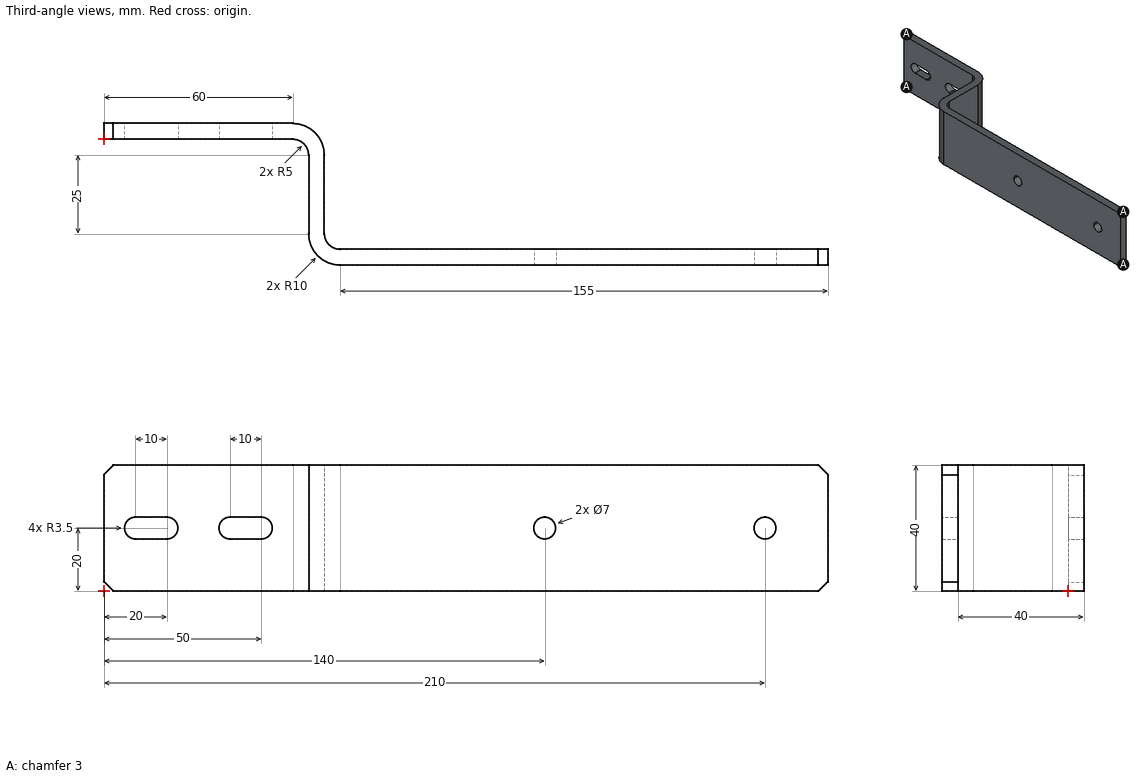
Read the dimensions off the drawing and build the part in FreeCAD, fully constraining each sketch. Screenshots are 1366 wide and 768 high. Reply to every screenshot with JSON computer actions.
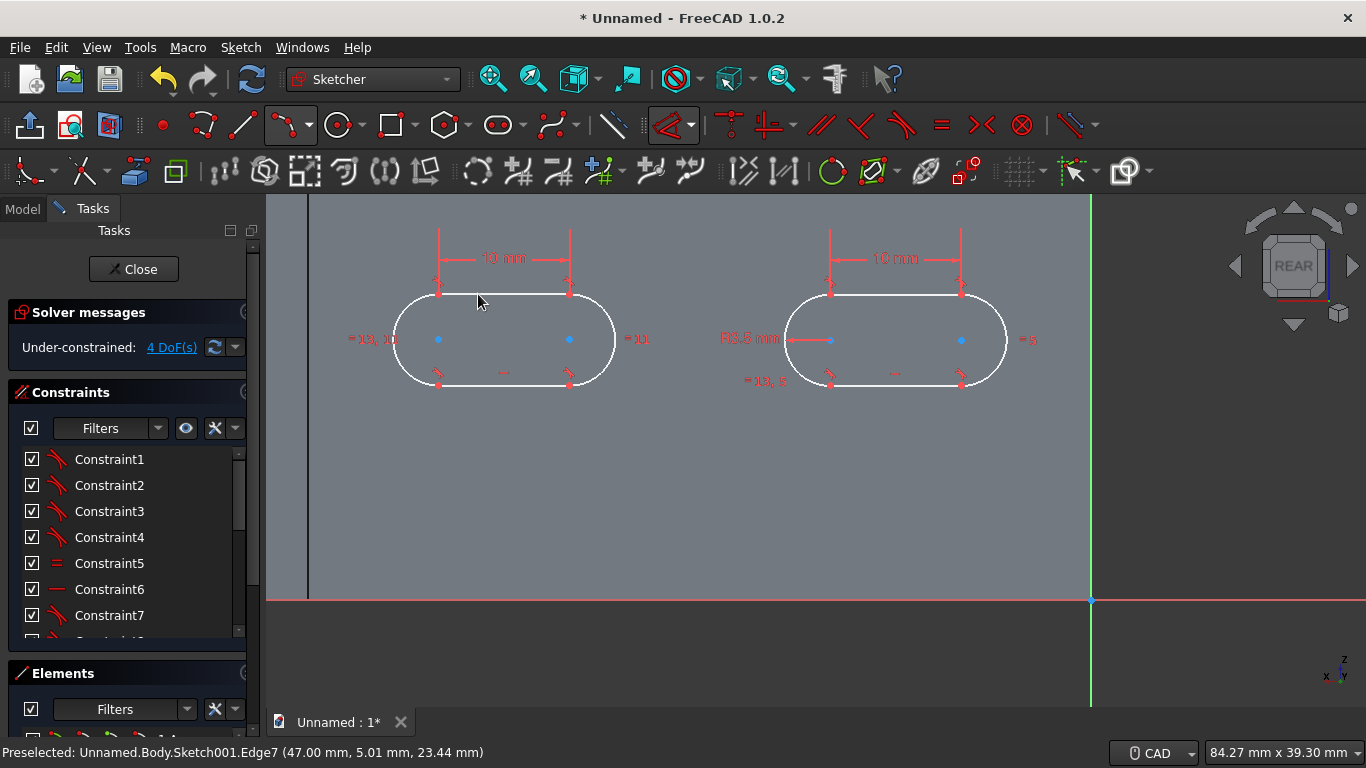
{"action": "left_click", "coordinate": [830, 295]}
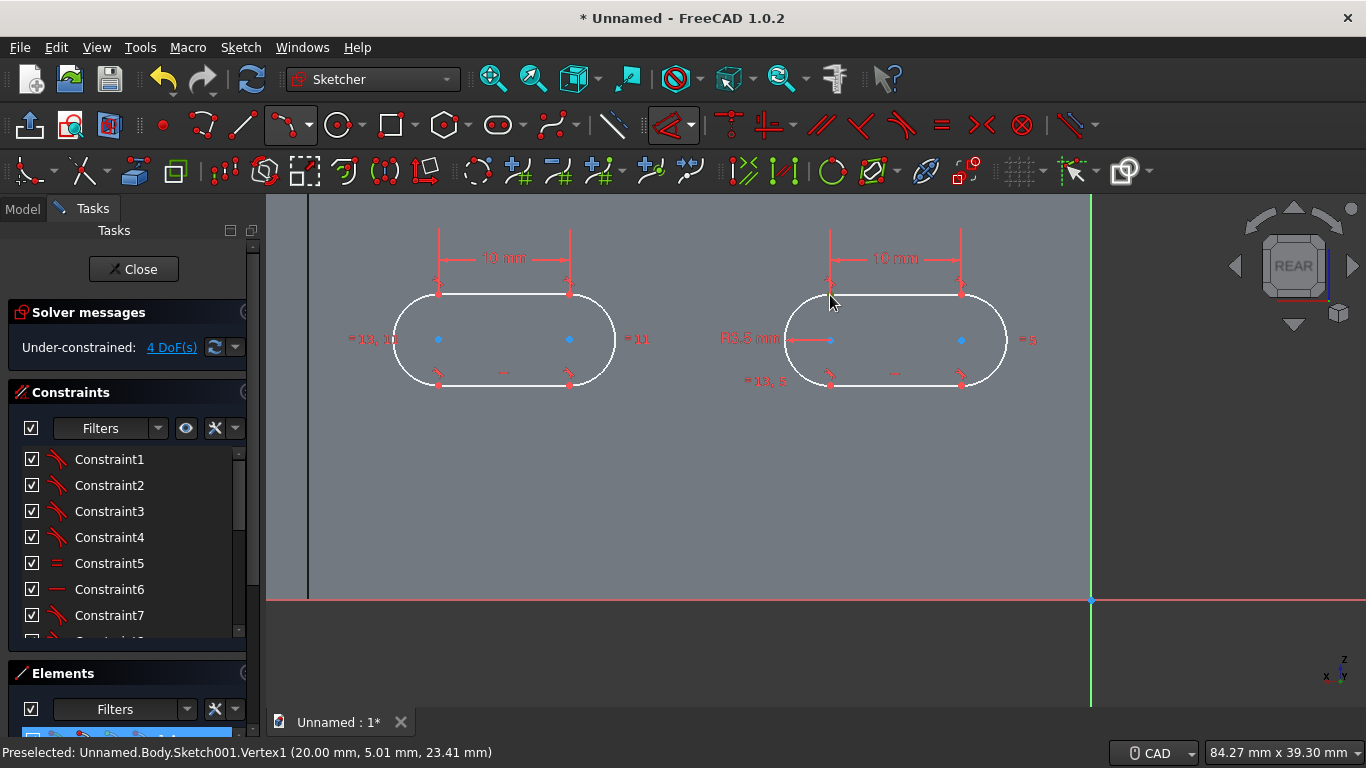
{"action": "left_click", "coordinate": [694, 126]}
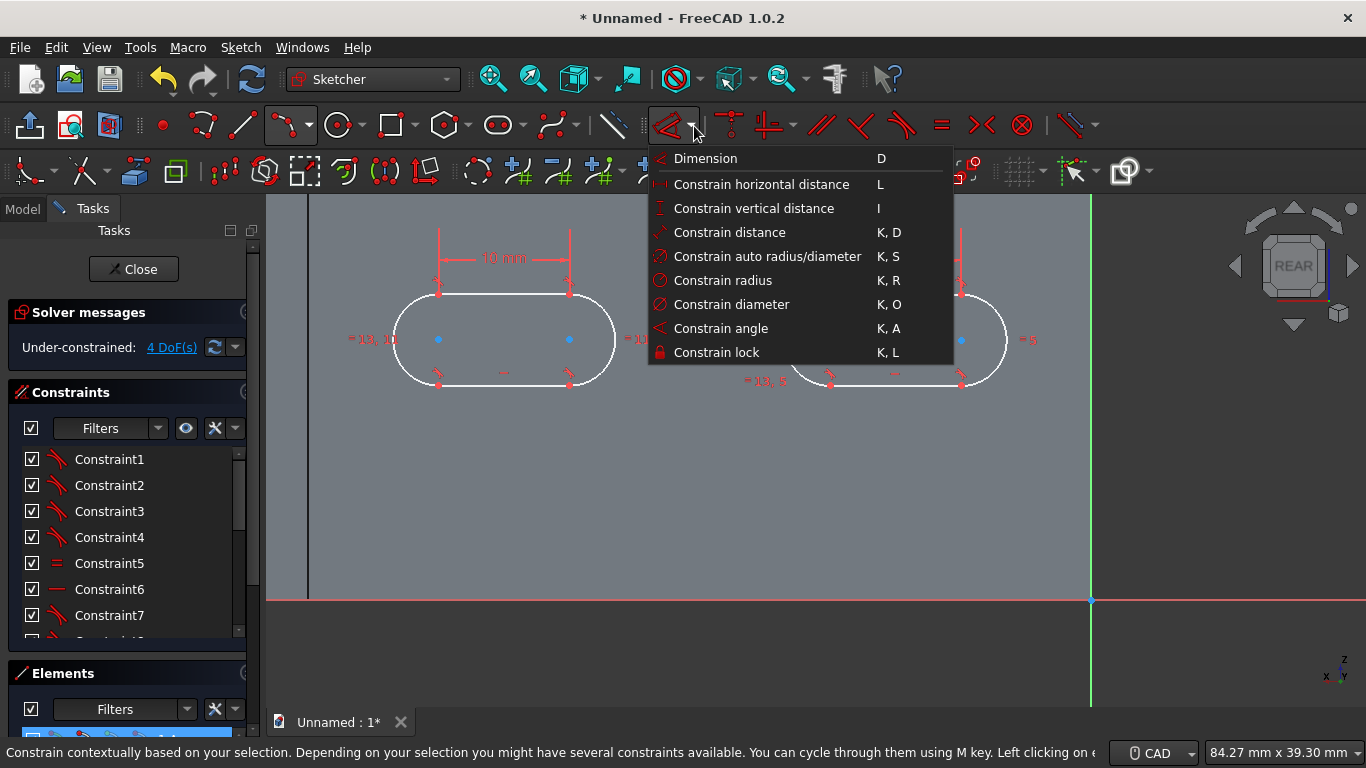
{"action": "left_click", "coordinate": [801, 184]}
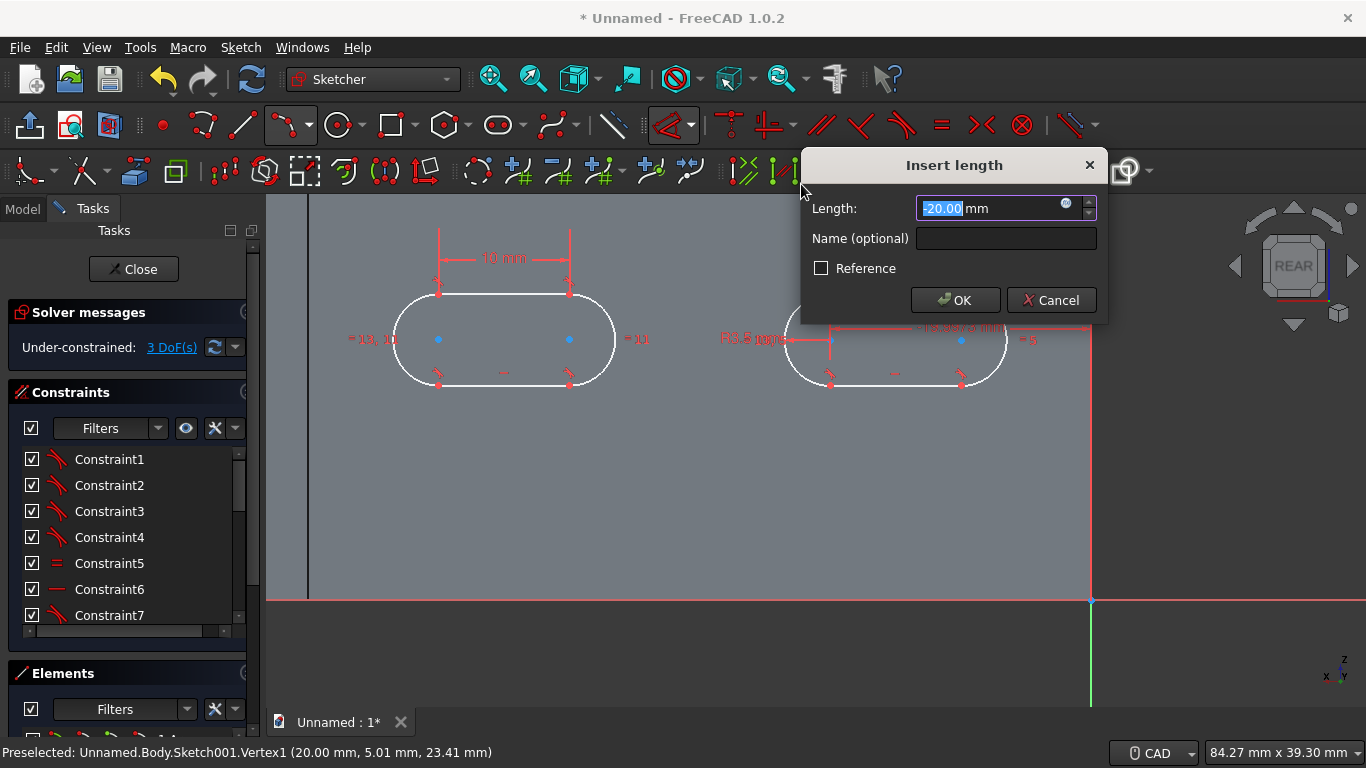
{"action": "type", "text": "-20"}
{"action": "key", "text": "Return"}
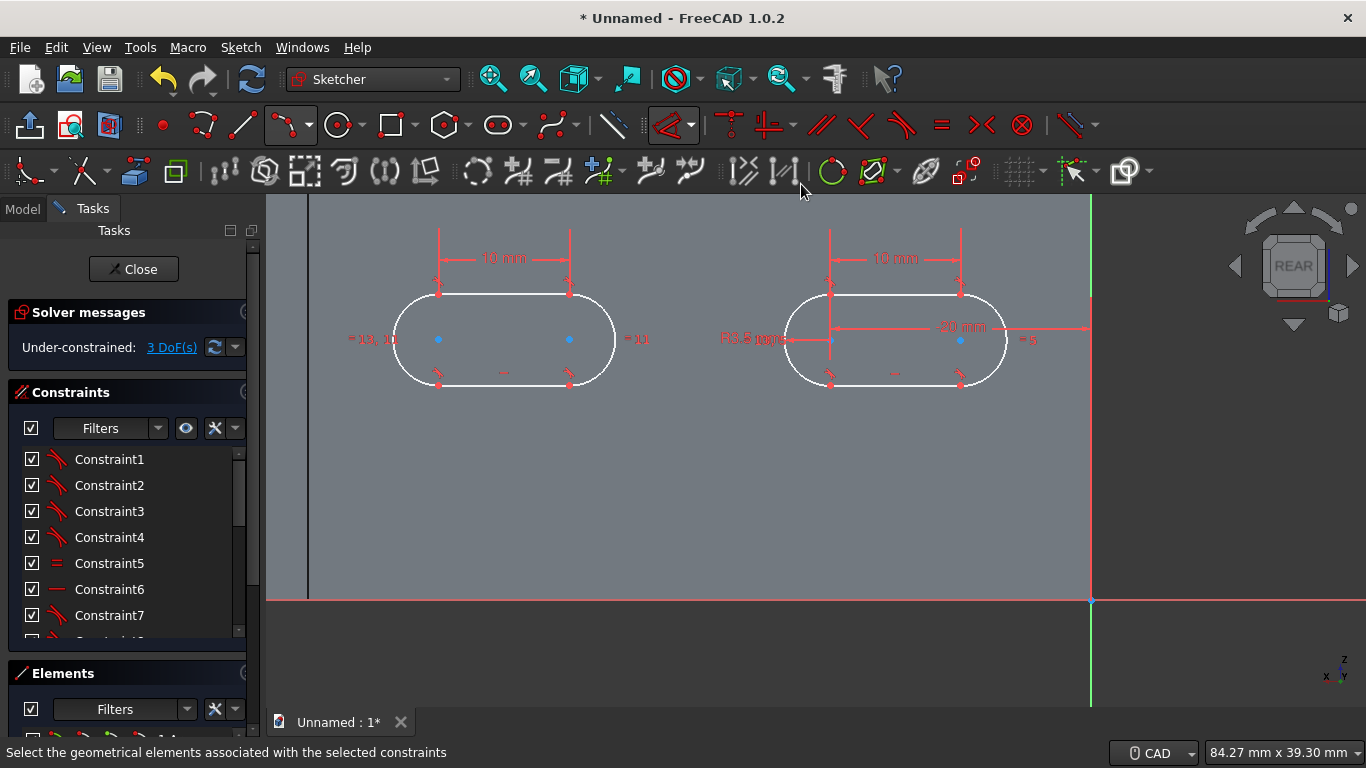
{"action": "left_click", "coordinate": [439, 294]}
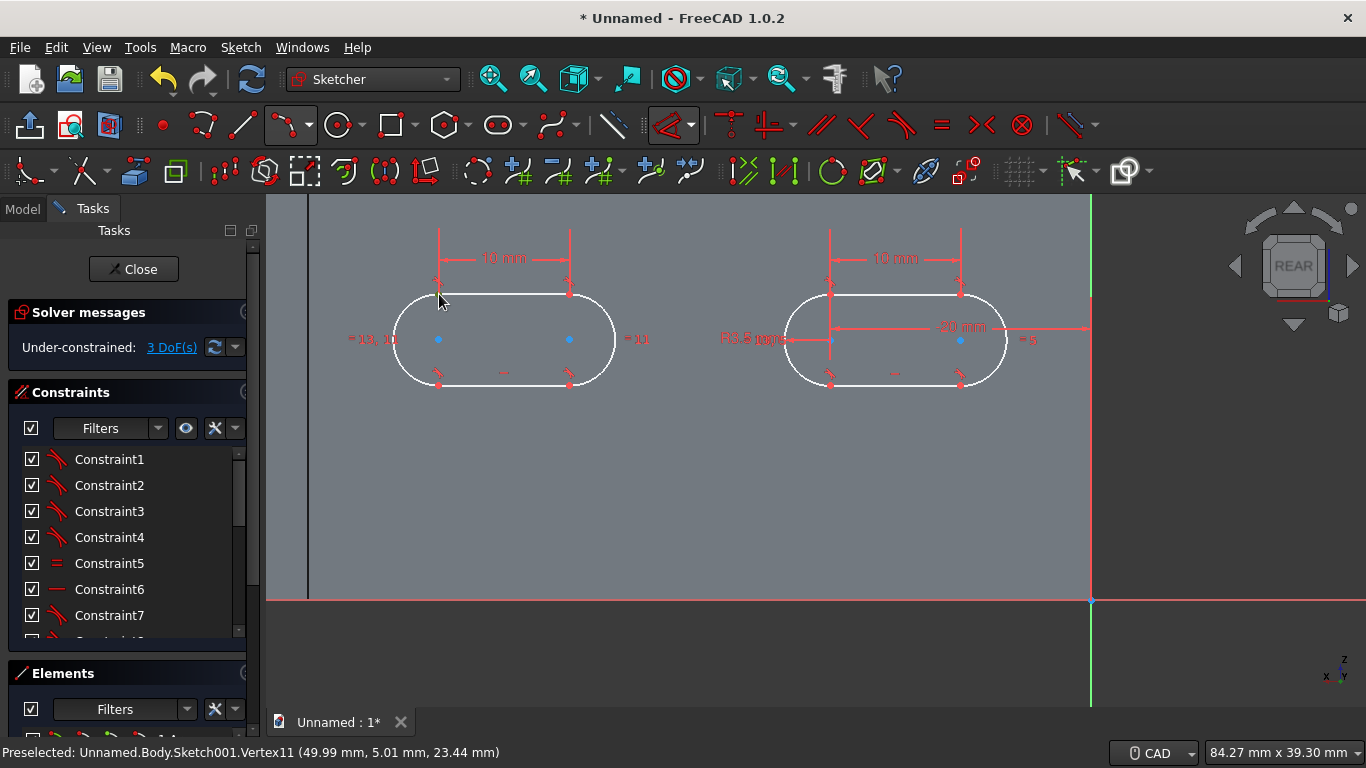
{"action": "left_click", "coordinate": [694, 126]}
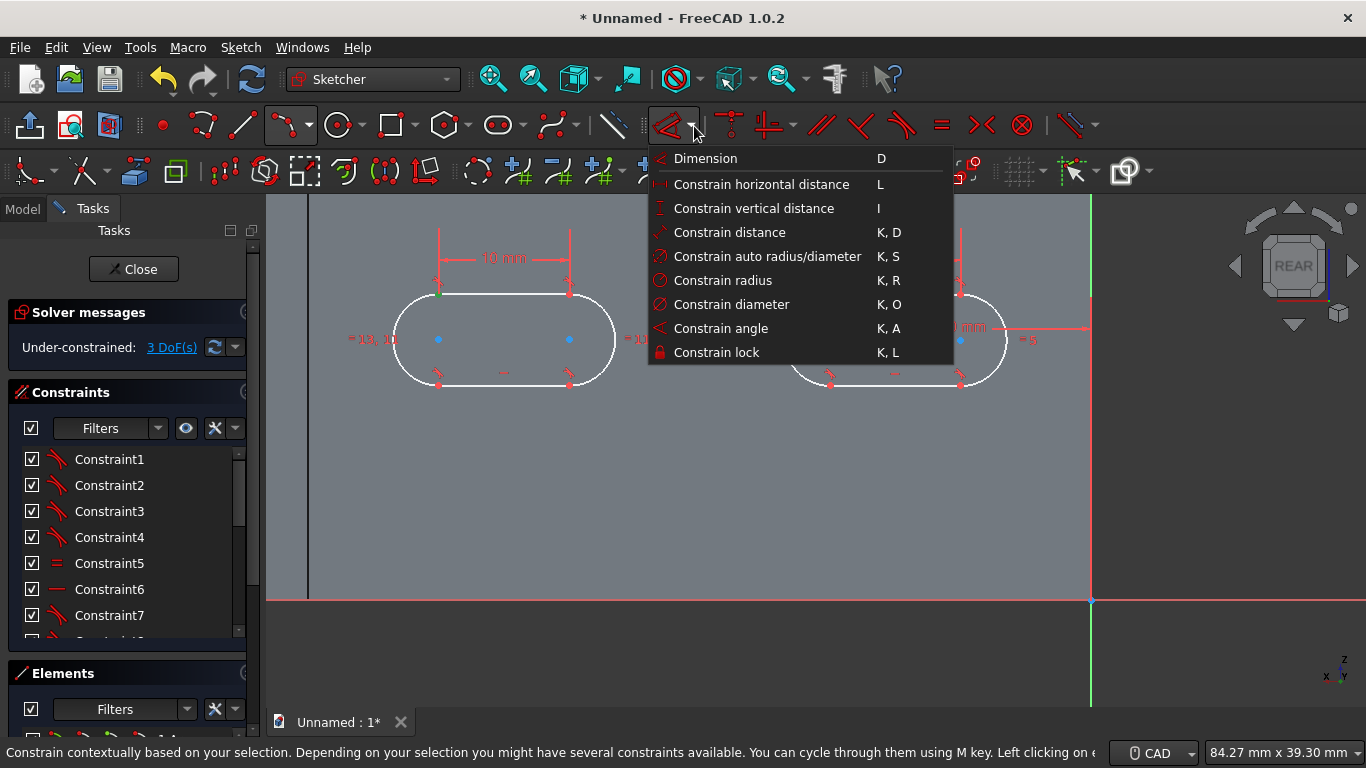
{"action": "left_click", "coordinate": [801, 184]}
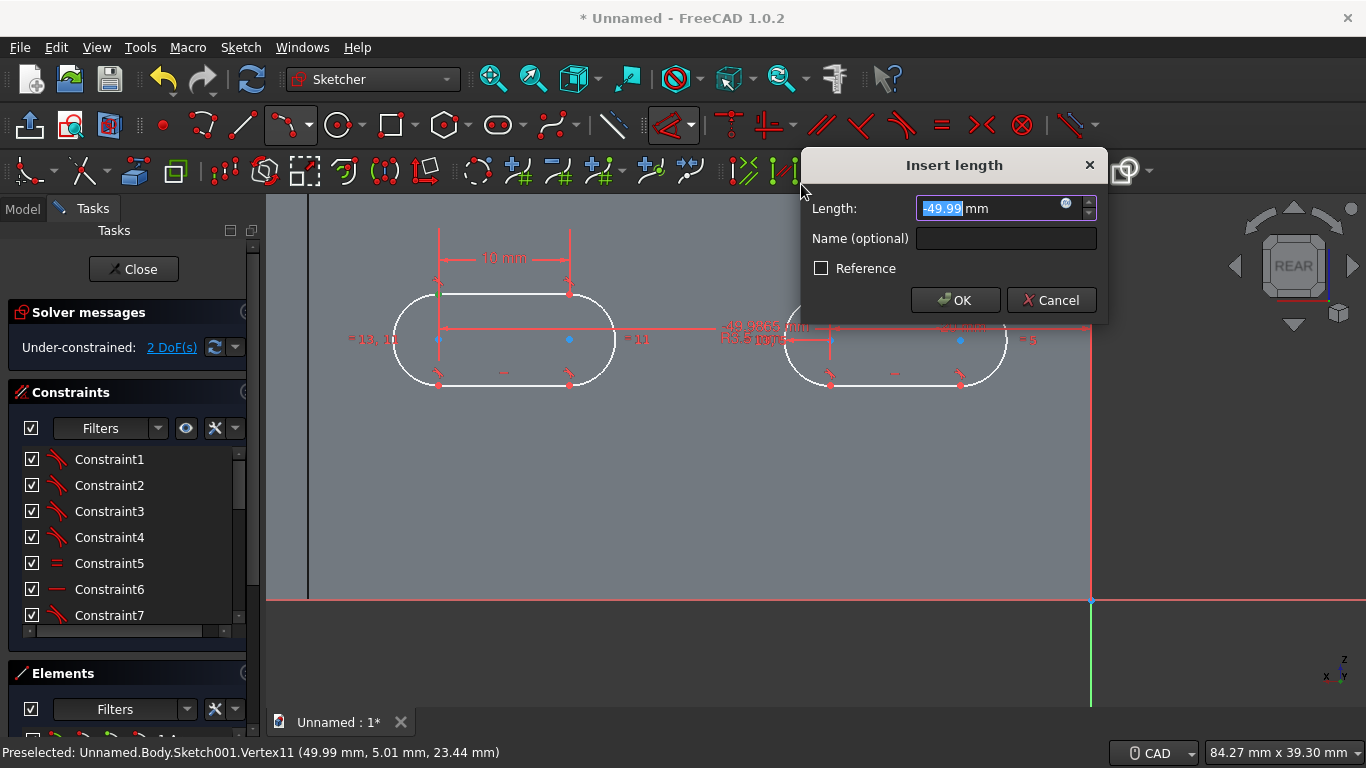
{"action": "type", "text": "-50"}
{"action": "key", "text": "Return"}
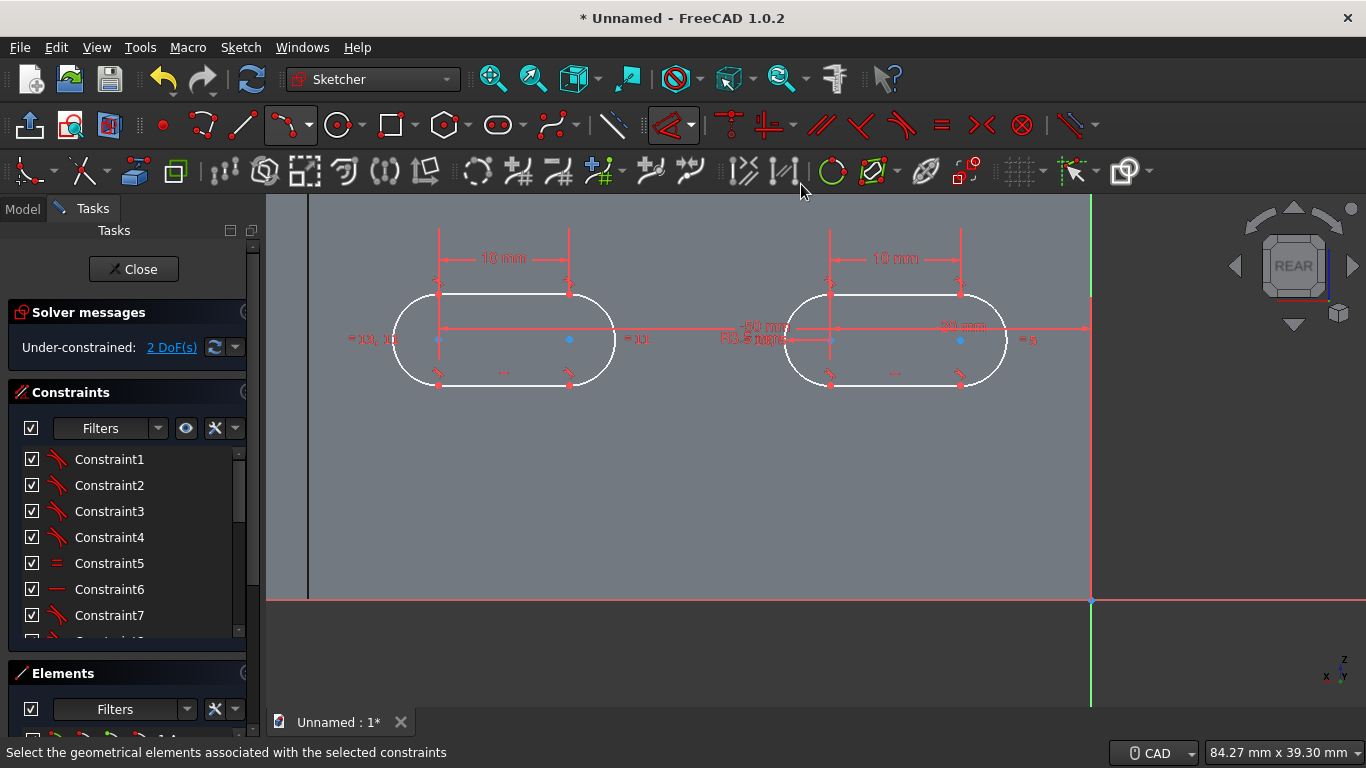
{"action": "left_click", "coordinate": [830, 340]}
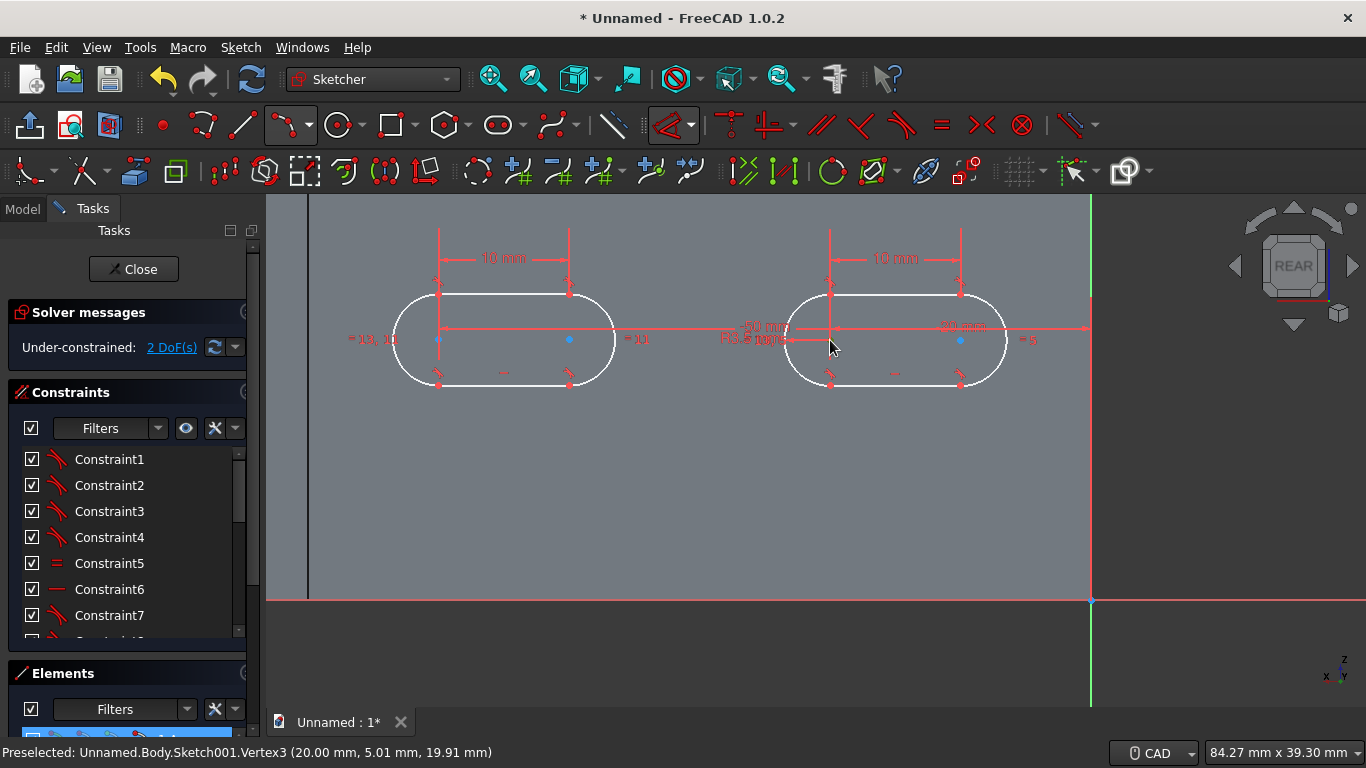
{"action": "key", "text": "i"}